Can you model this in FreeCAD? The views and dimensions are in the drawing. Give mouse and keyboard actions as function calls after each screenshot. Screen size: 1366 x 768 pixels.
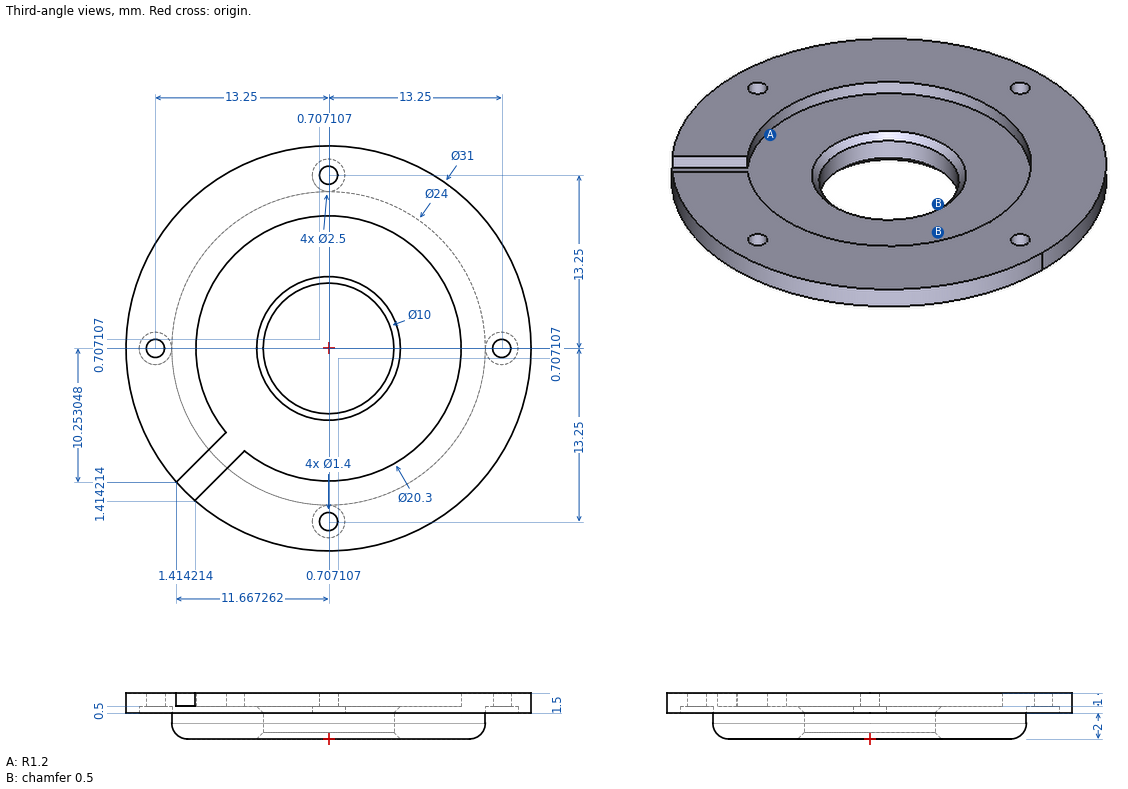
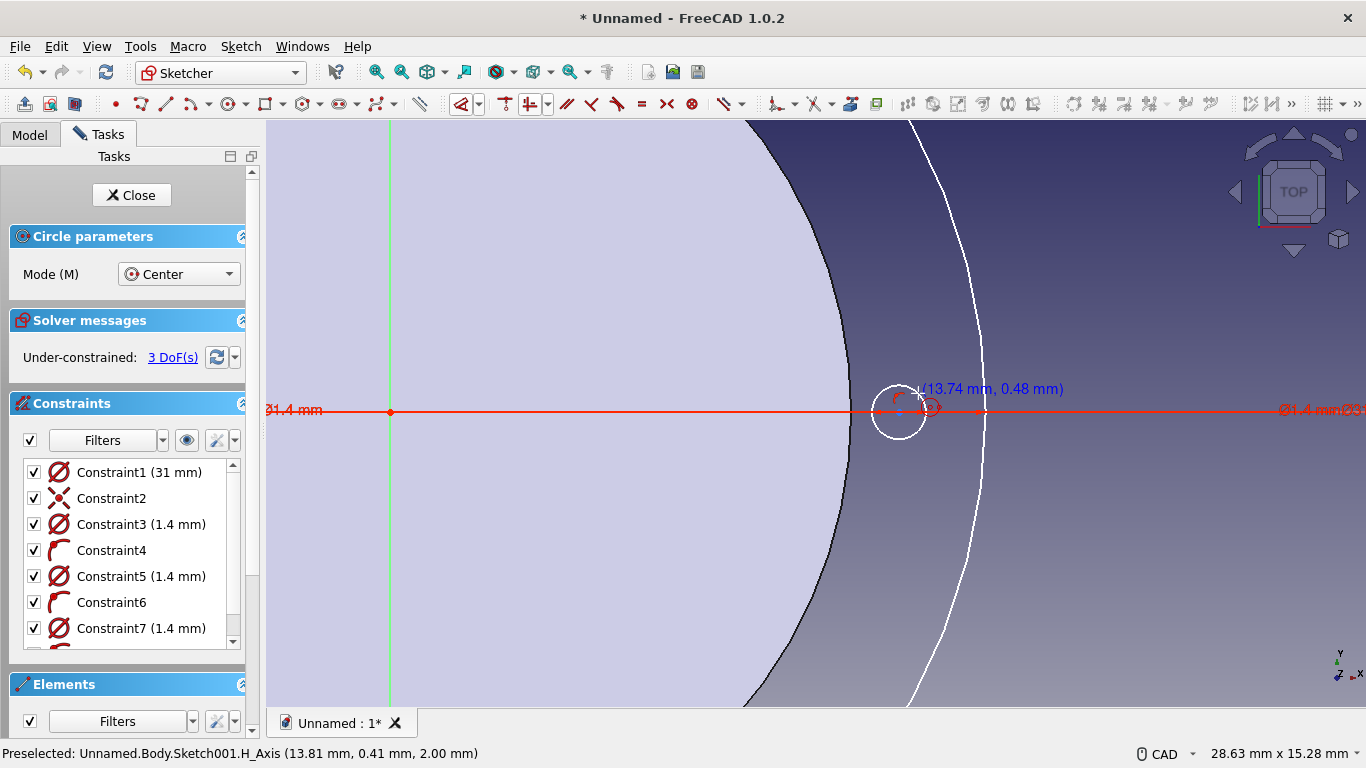
scroll(902, 414, down, 6)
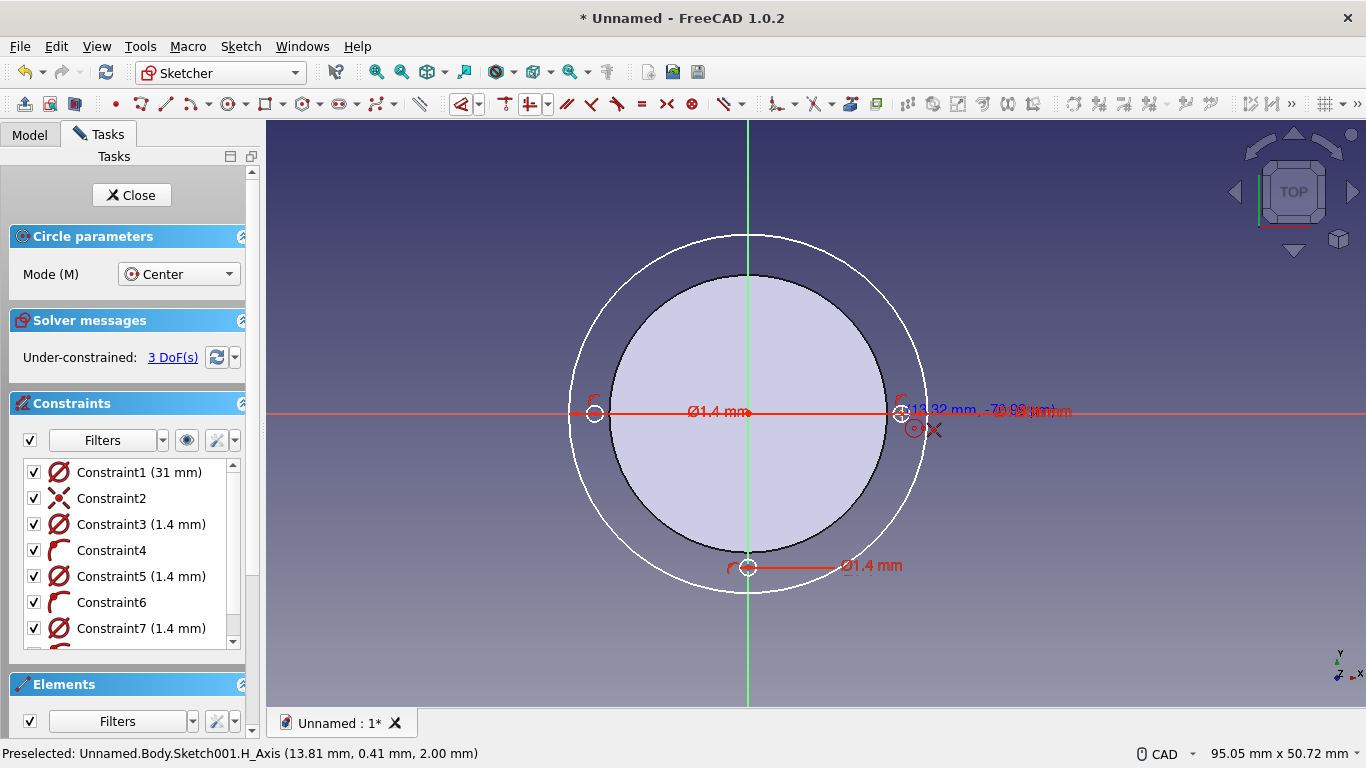
scroll(748, 260, up, 6)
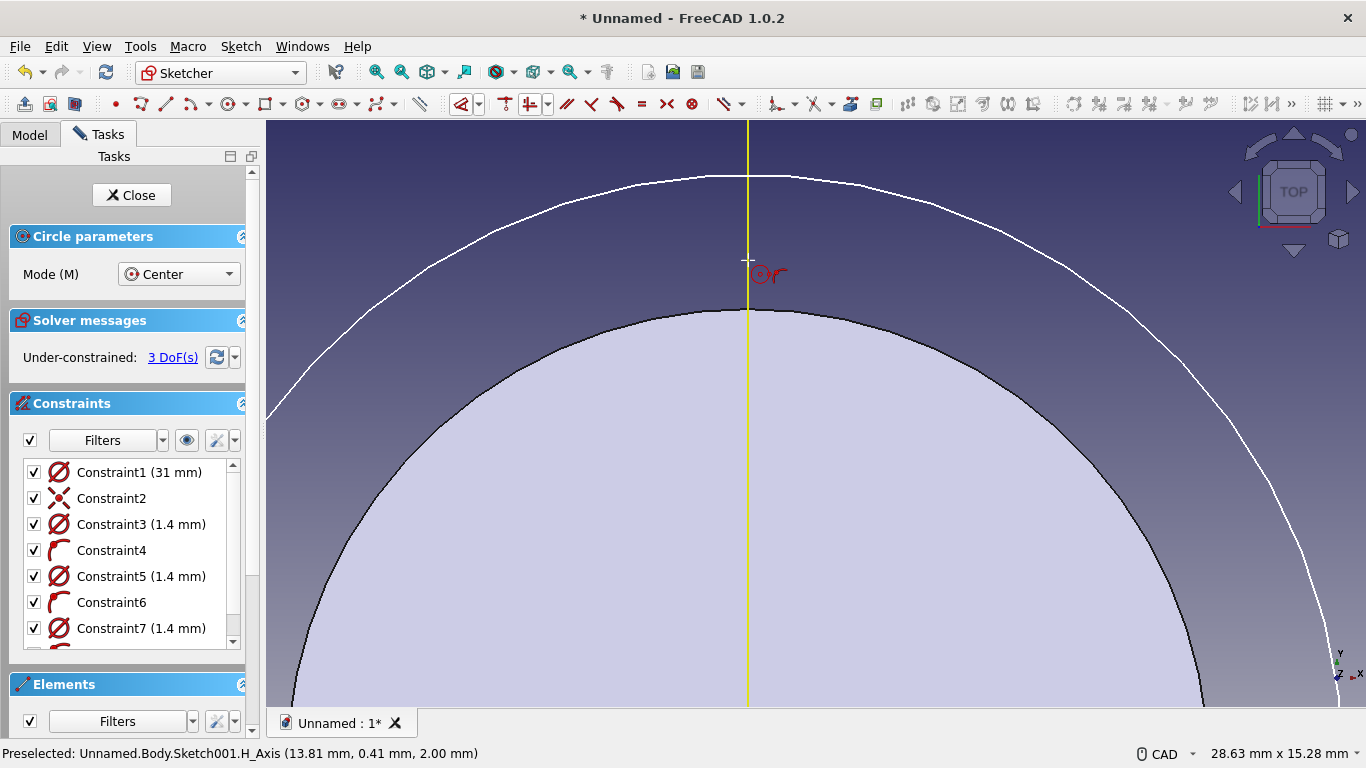
click(748, 261)
move(767, 242)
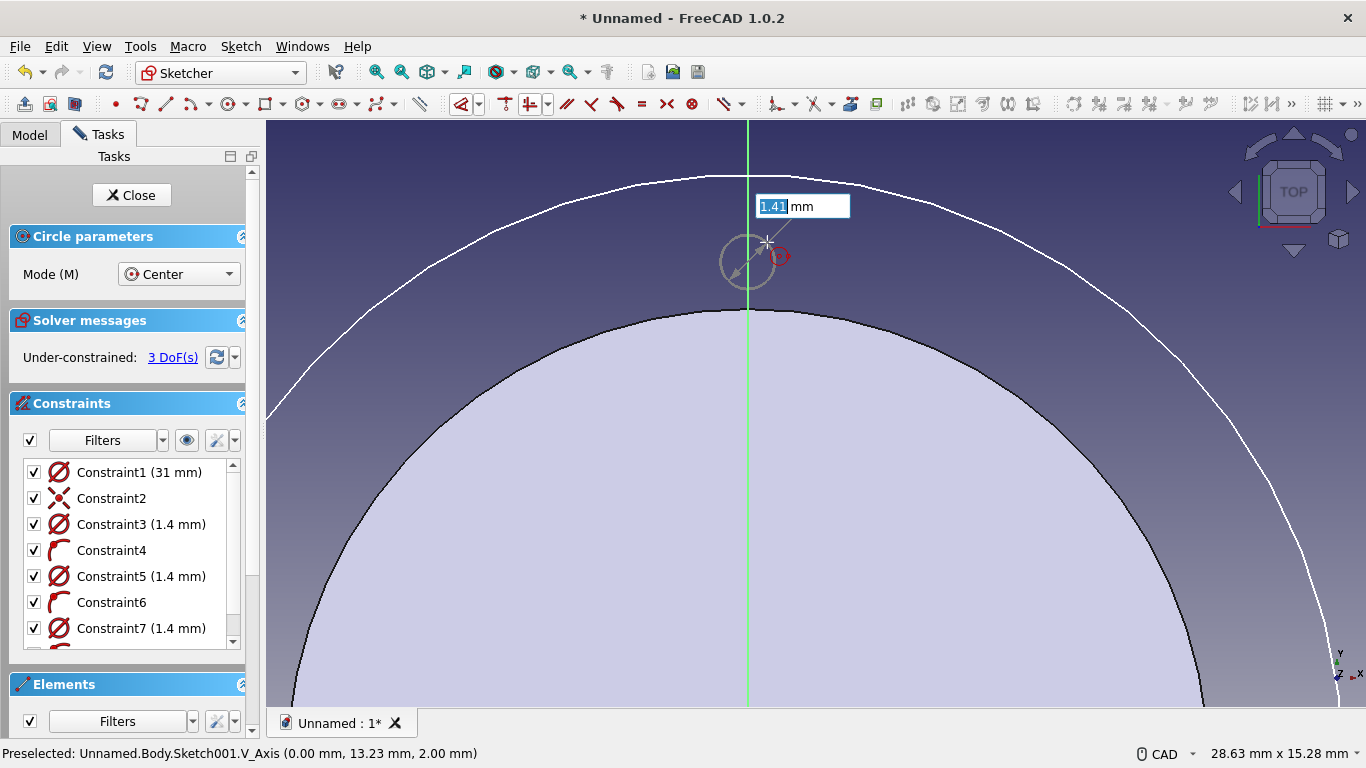
text(1.4)
key(Return)
key(Escape)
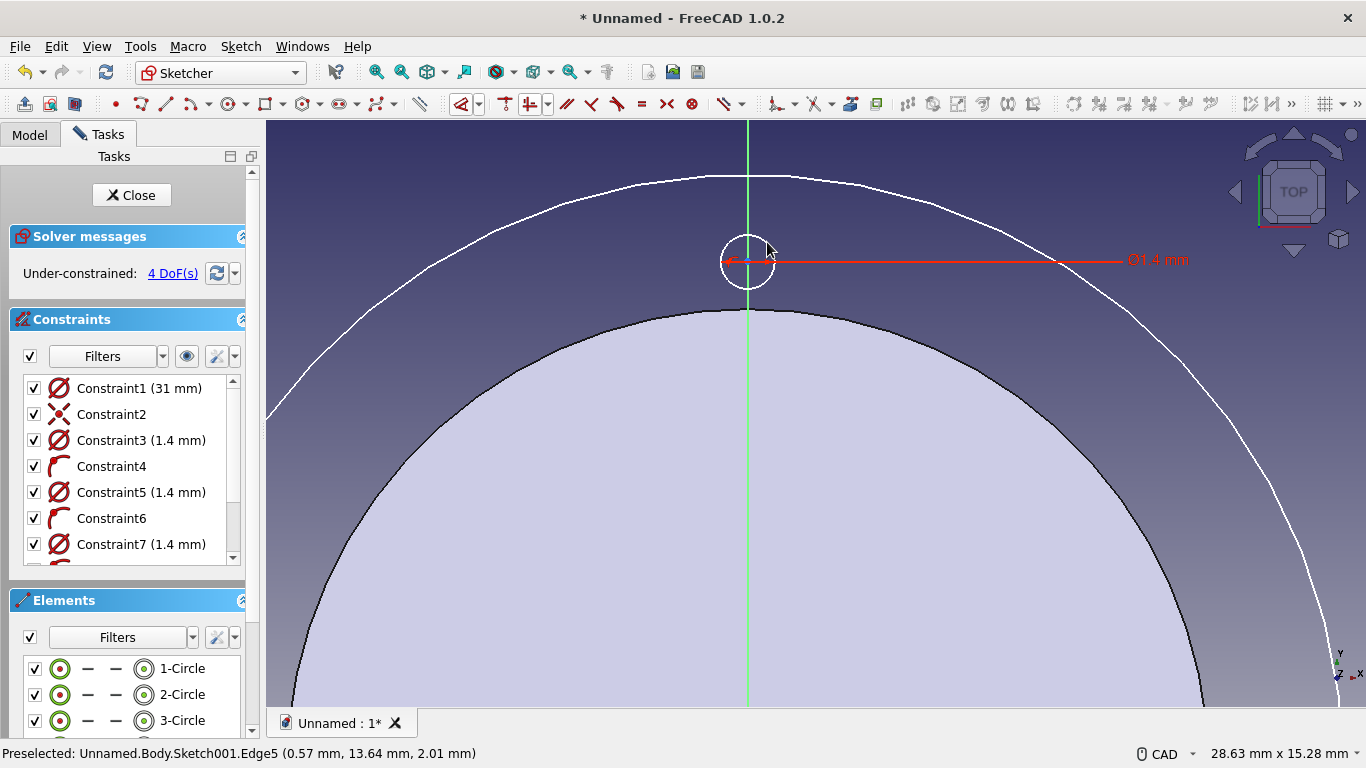
click(460, 104)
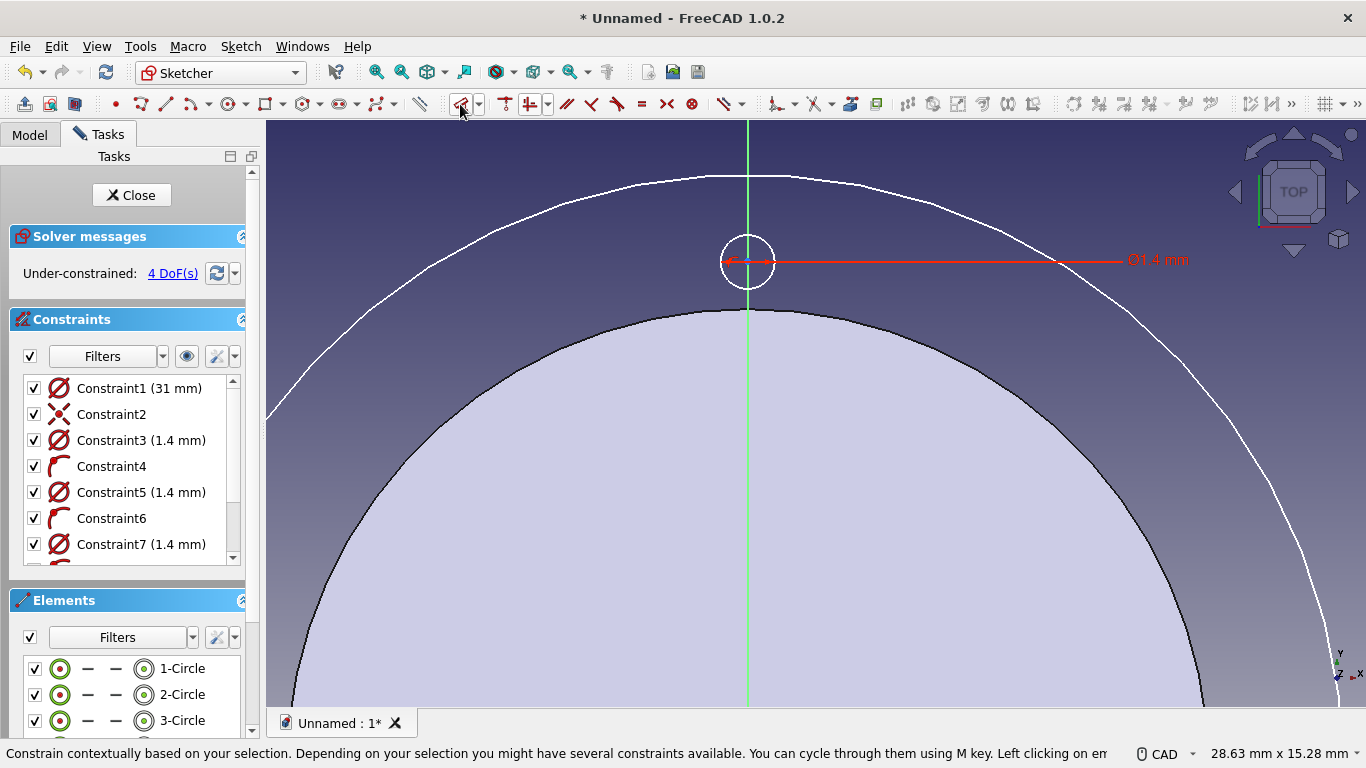
scroll(747, 260, down, 6)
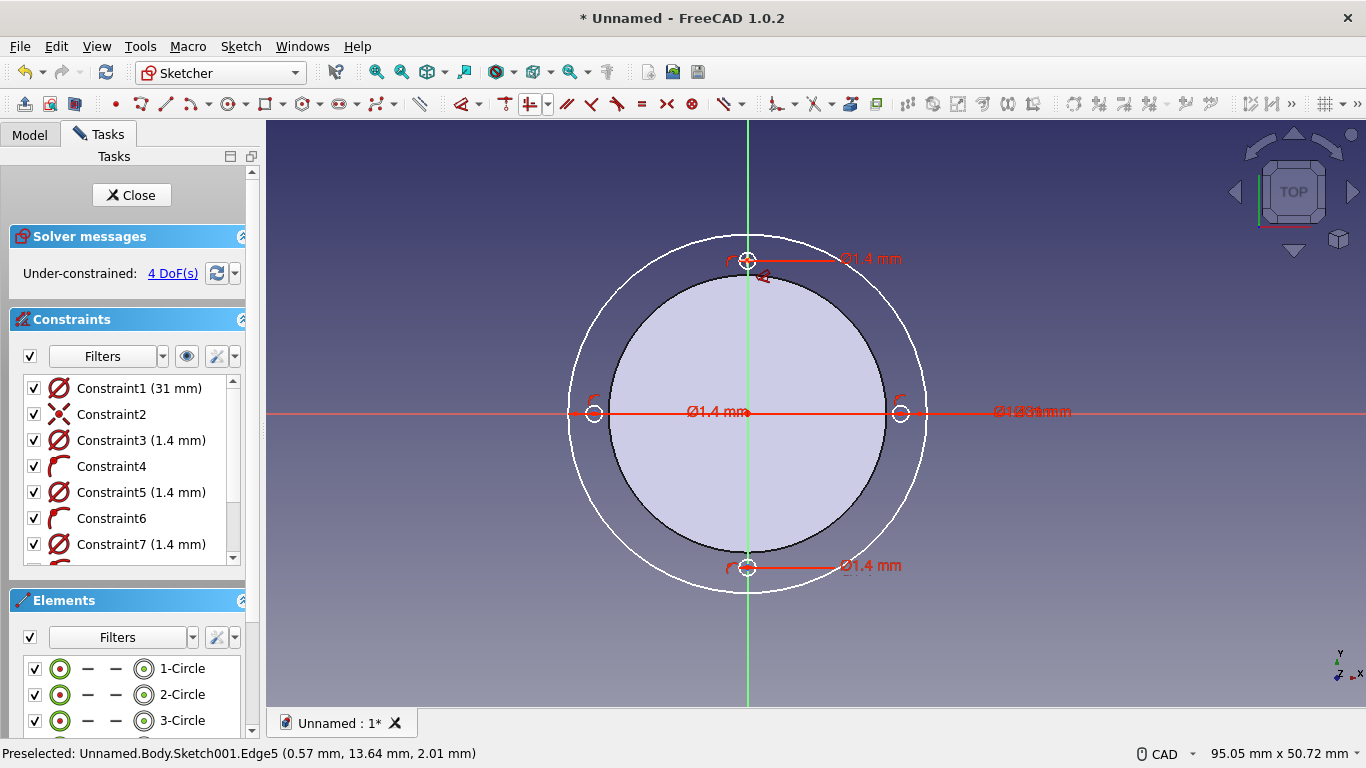
click(748, 568)
click(782, 491)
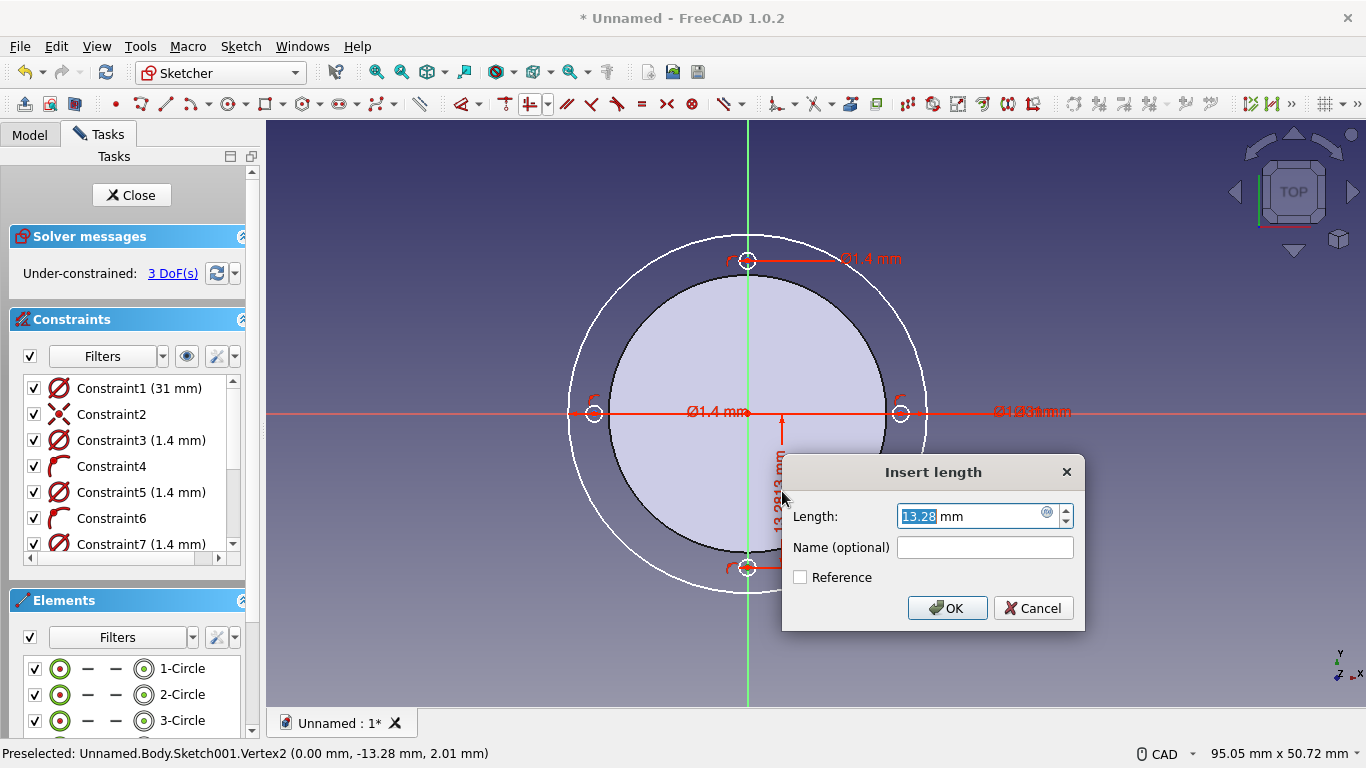
text(13.25)
key(Return)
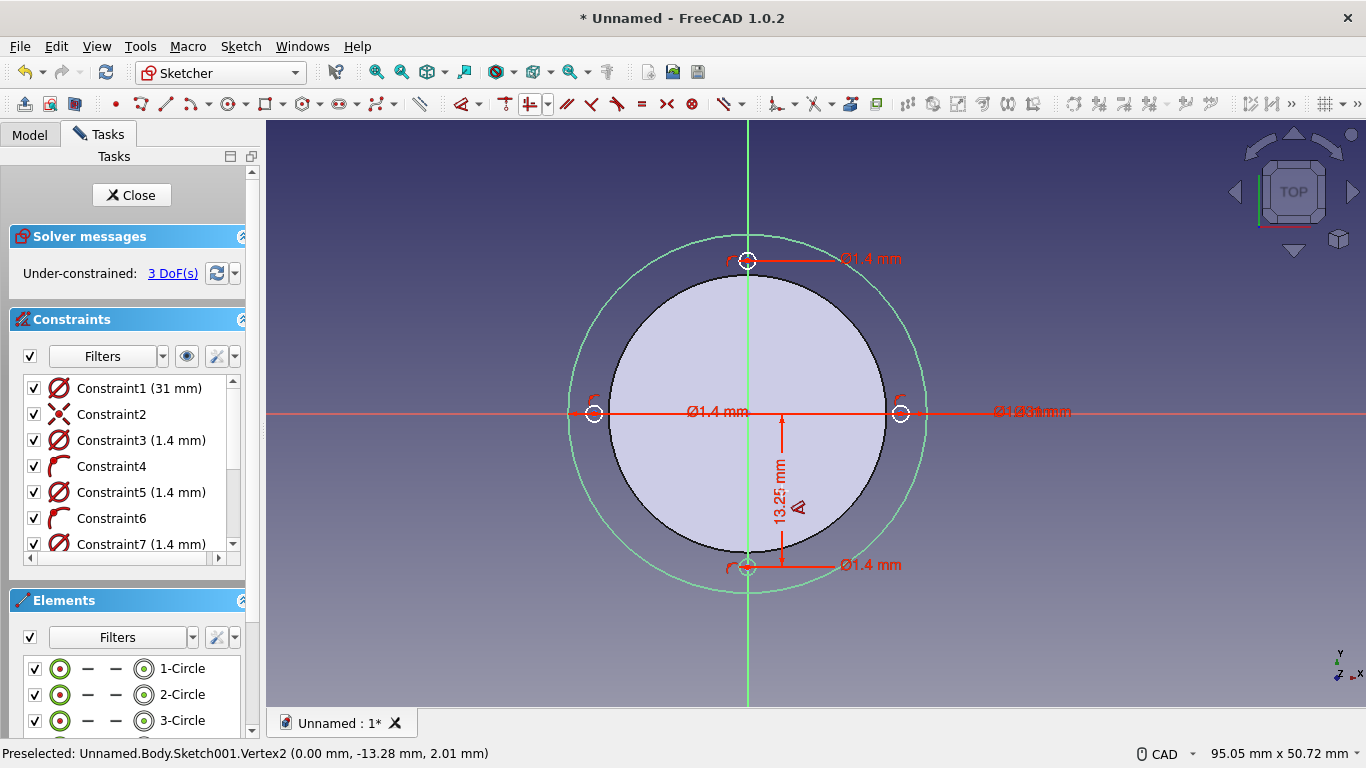
click(594, 414)
click(671, 448)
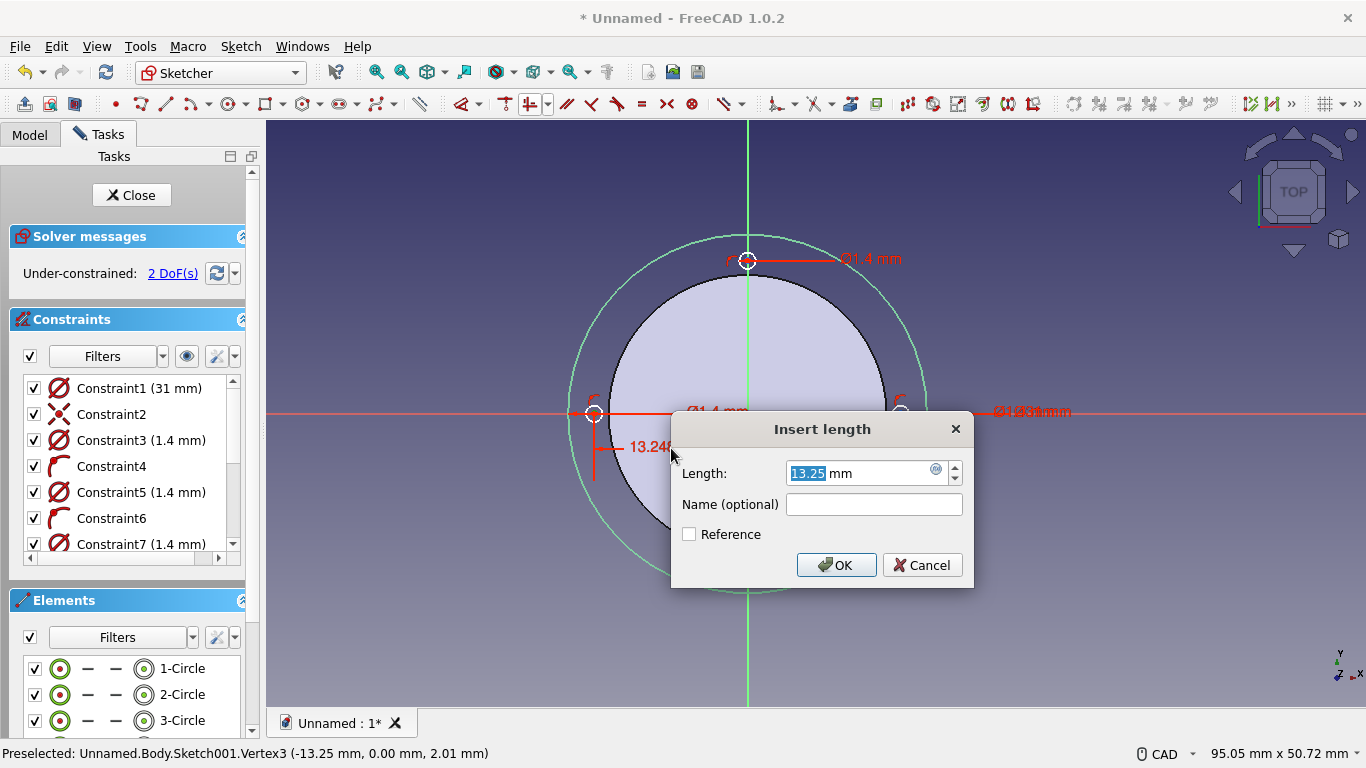
text(13.25)
key(Return)